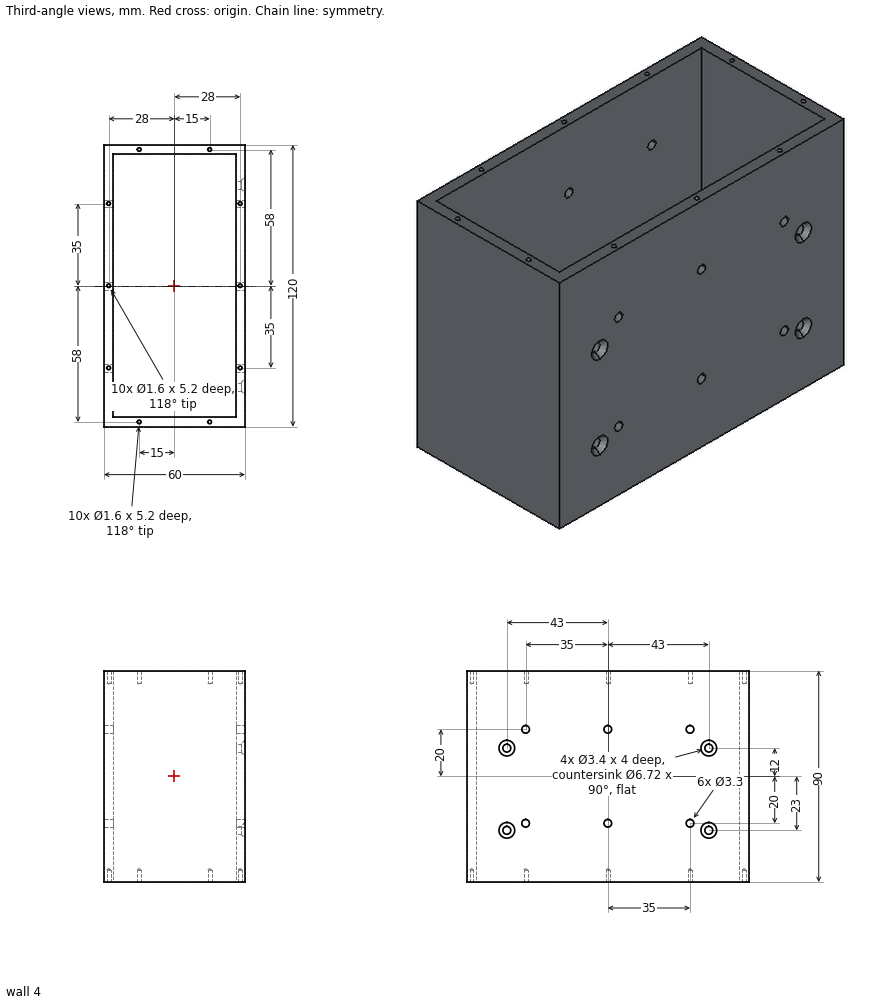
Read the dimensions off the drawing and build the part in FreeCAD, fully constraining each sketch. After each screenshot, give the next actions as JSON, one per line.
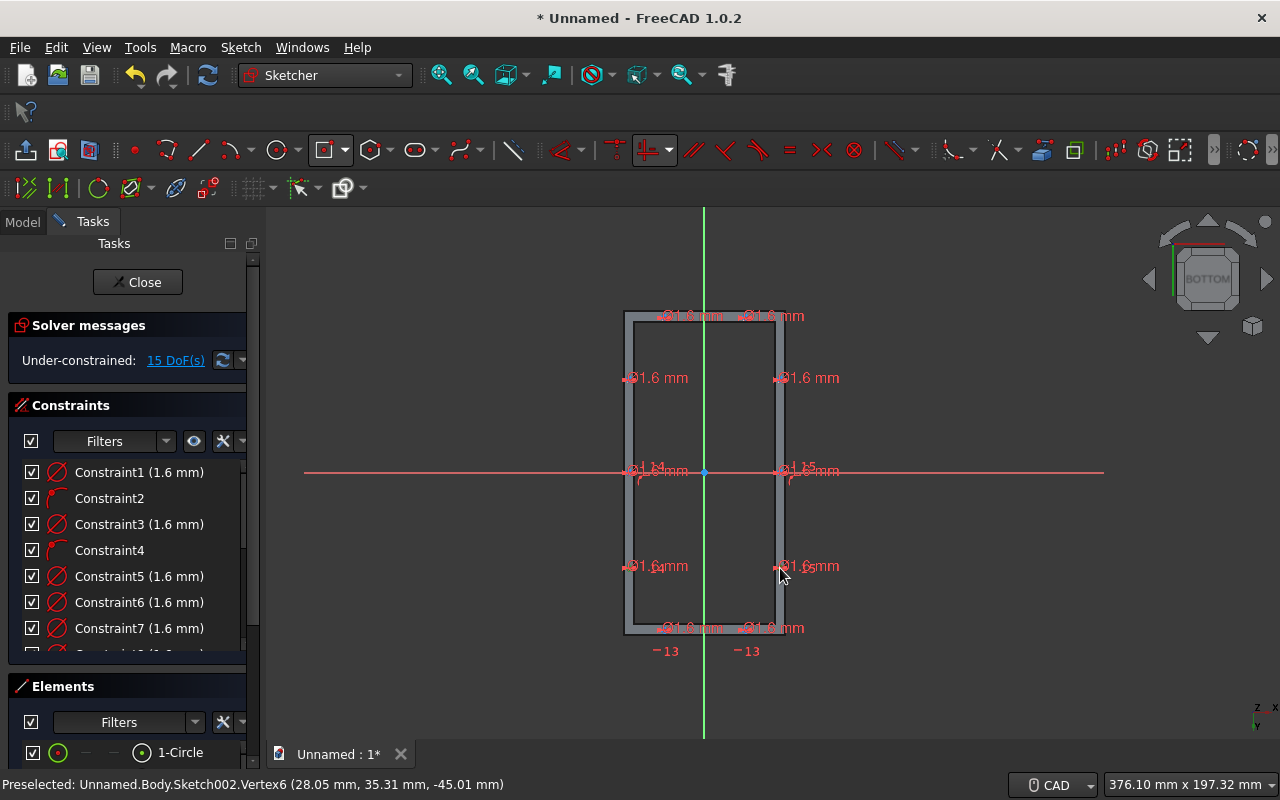
{"action": "left_click", "coordinate": [672, 150]}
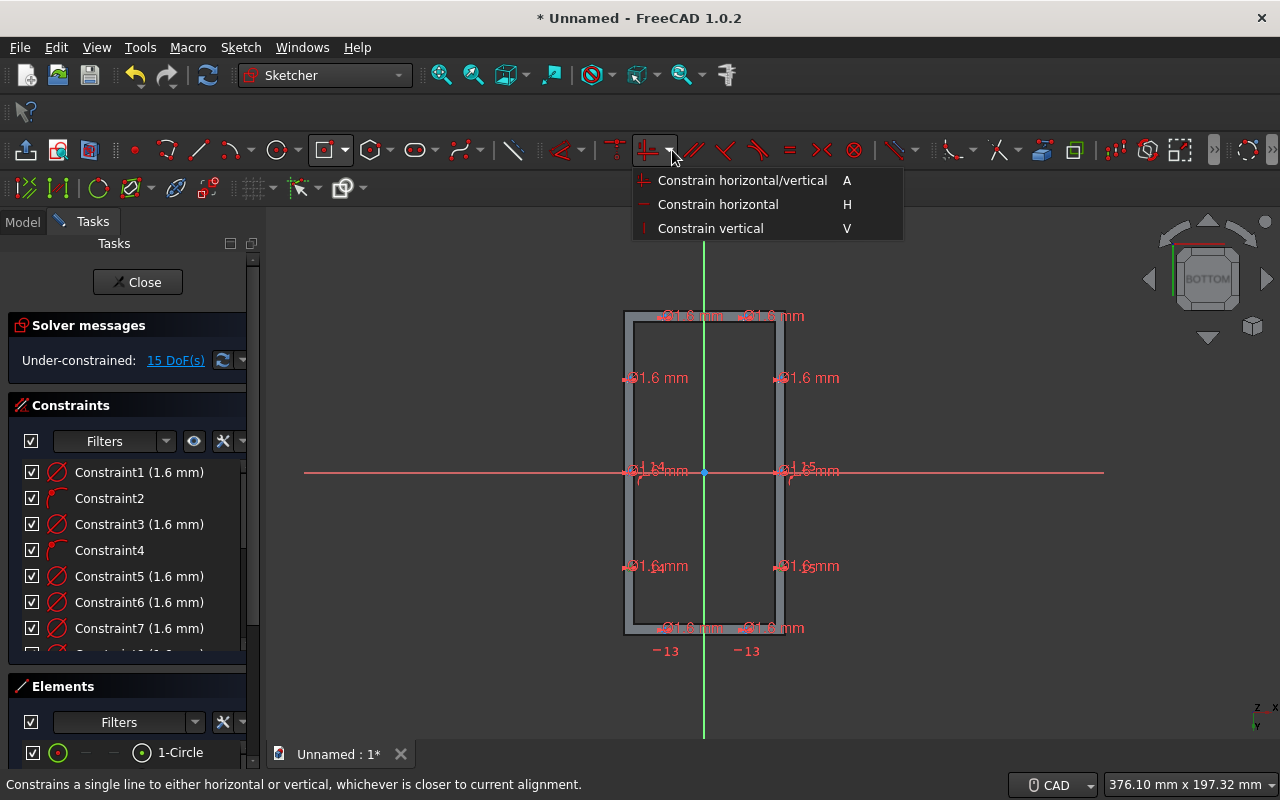
{"action": "left_click", "coordinate": [768, 204]}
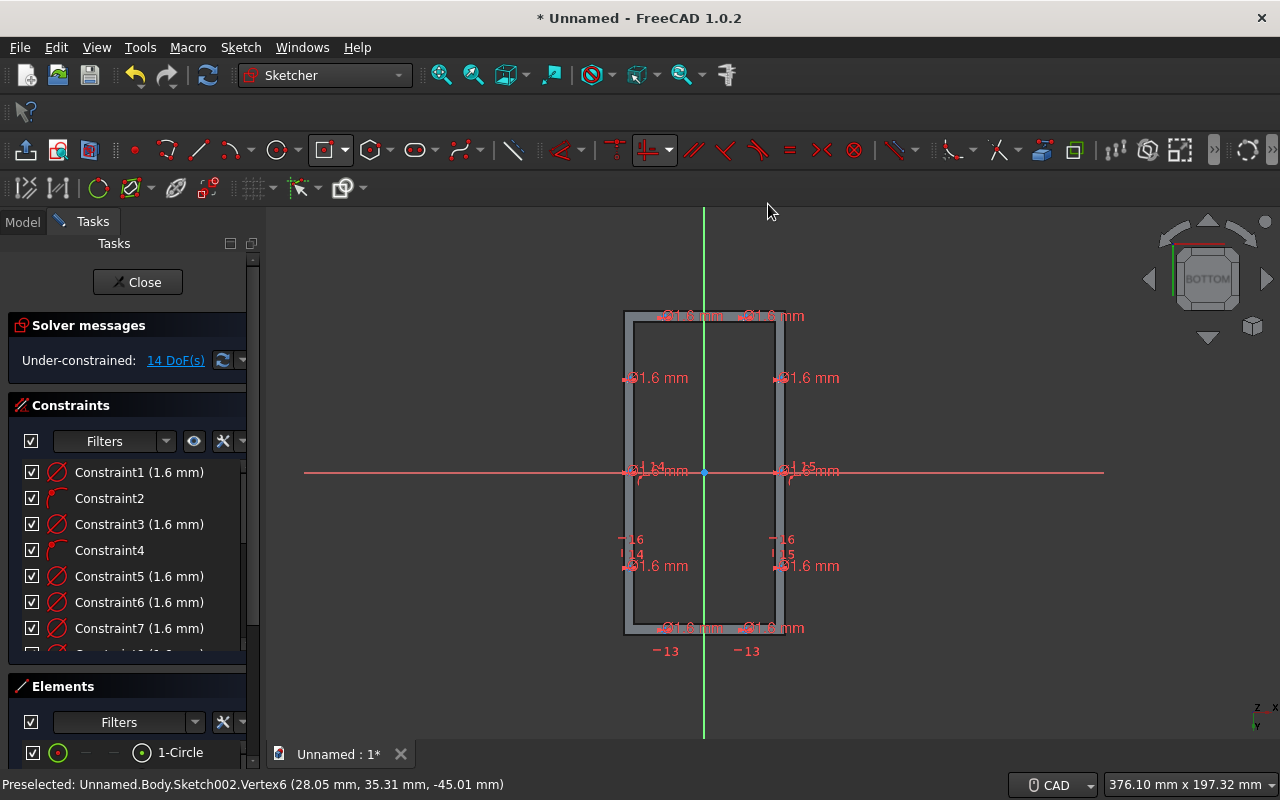
{"action": "left_click", "coordinate": [780, 473]}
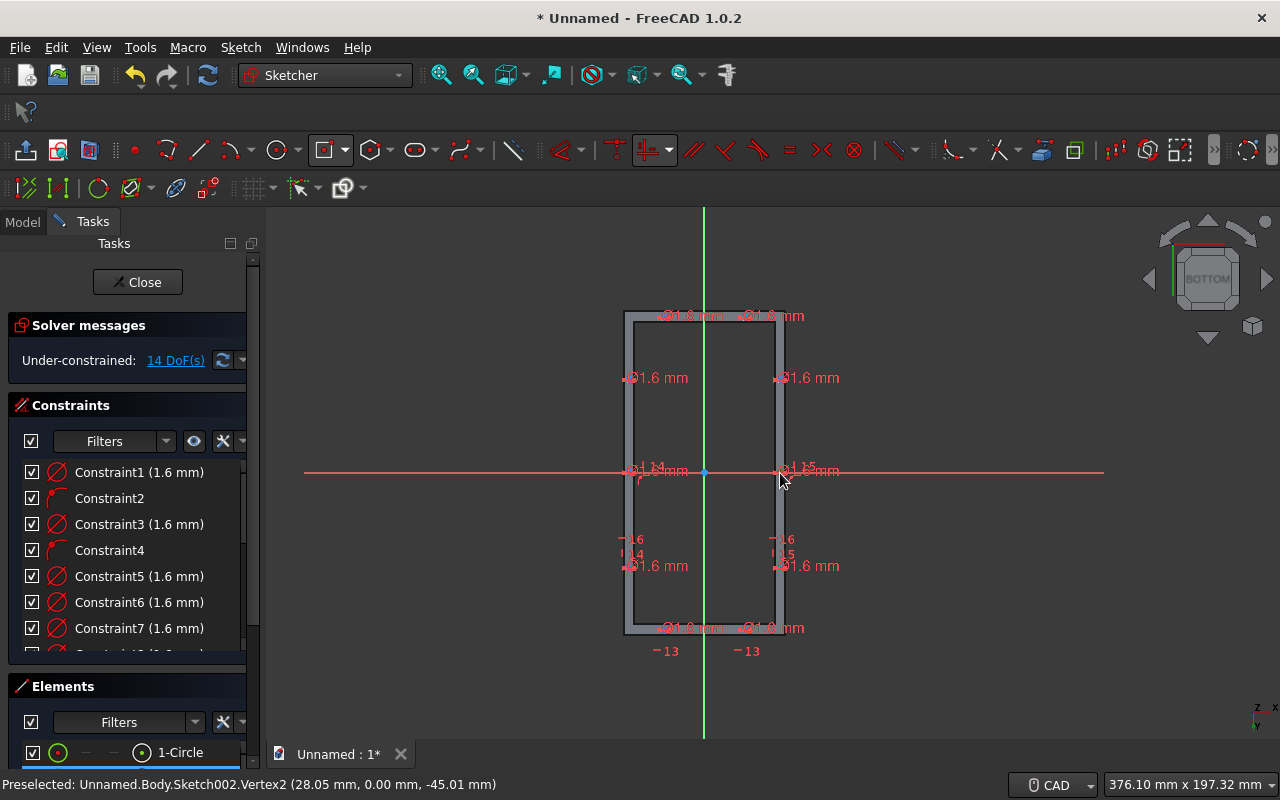
{"action": "left_click", "coordinate": [780, 380]}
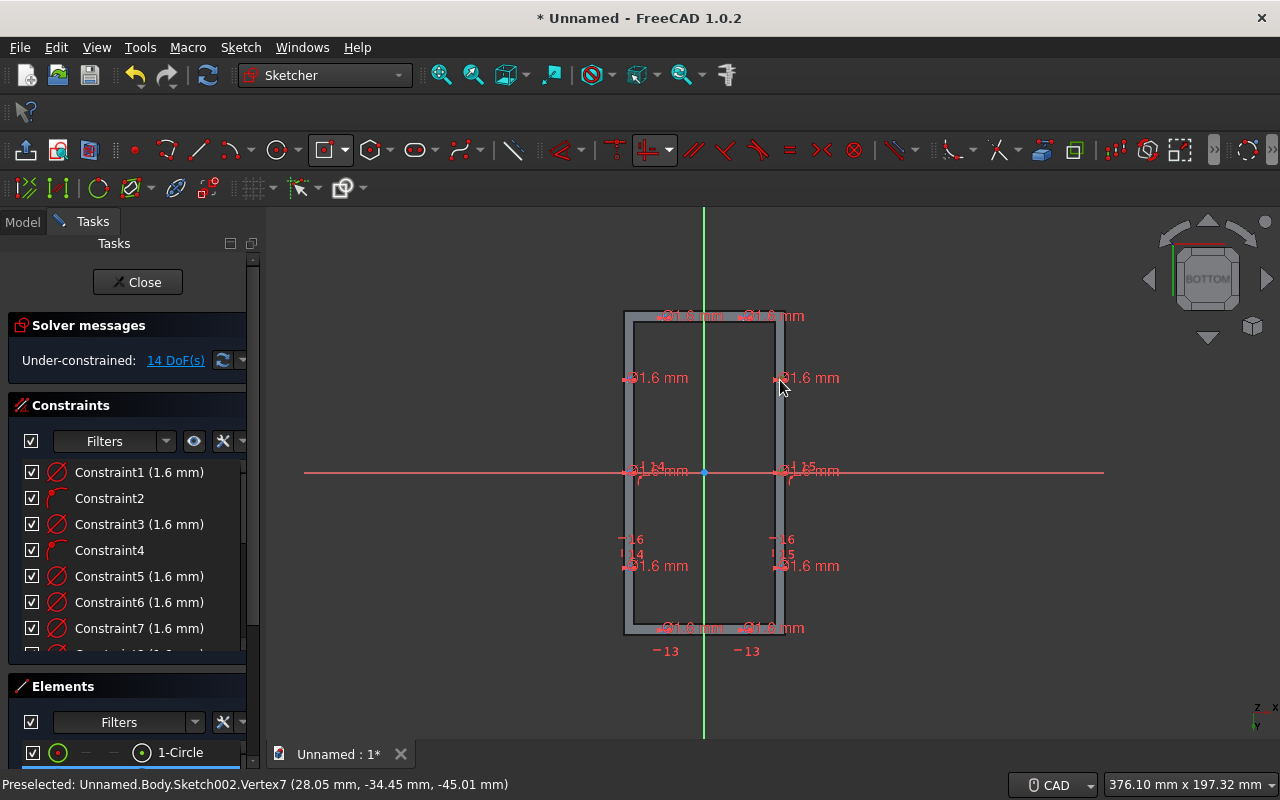
{"action": "left_click", "coordinate": [672, 150]}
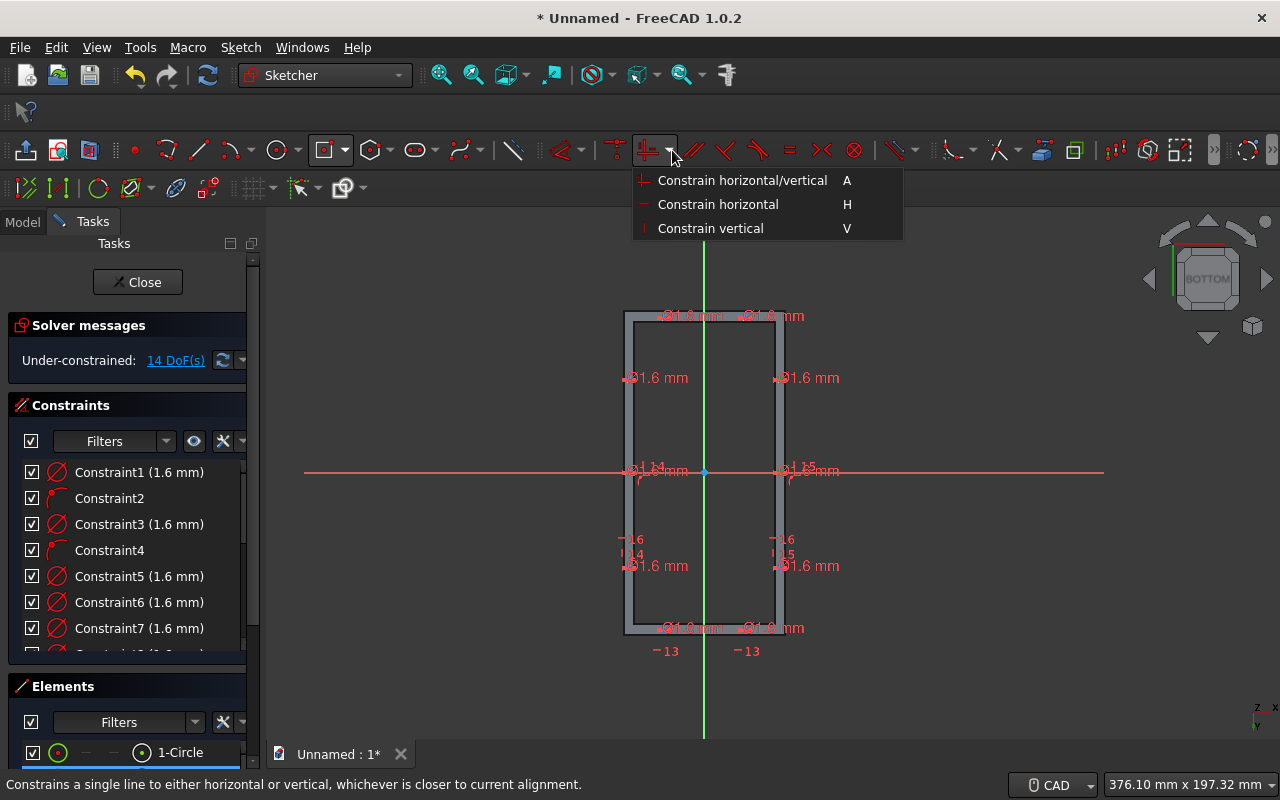
{"action": "left_click", "coordinate": [768, 228]}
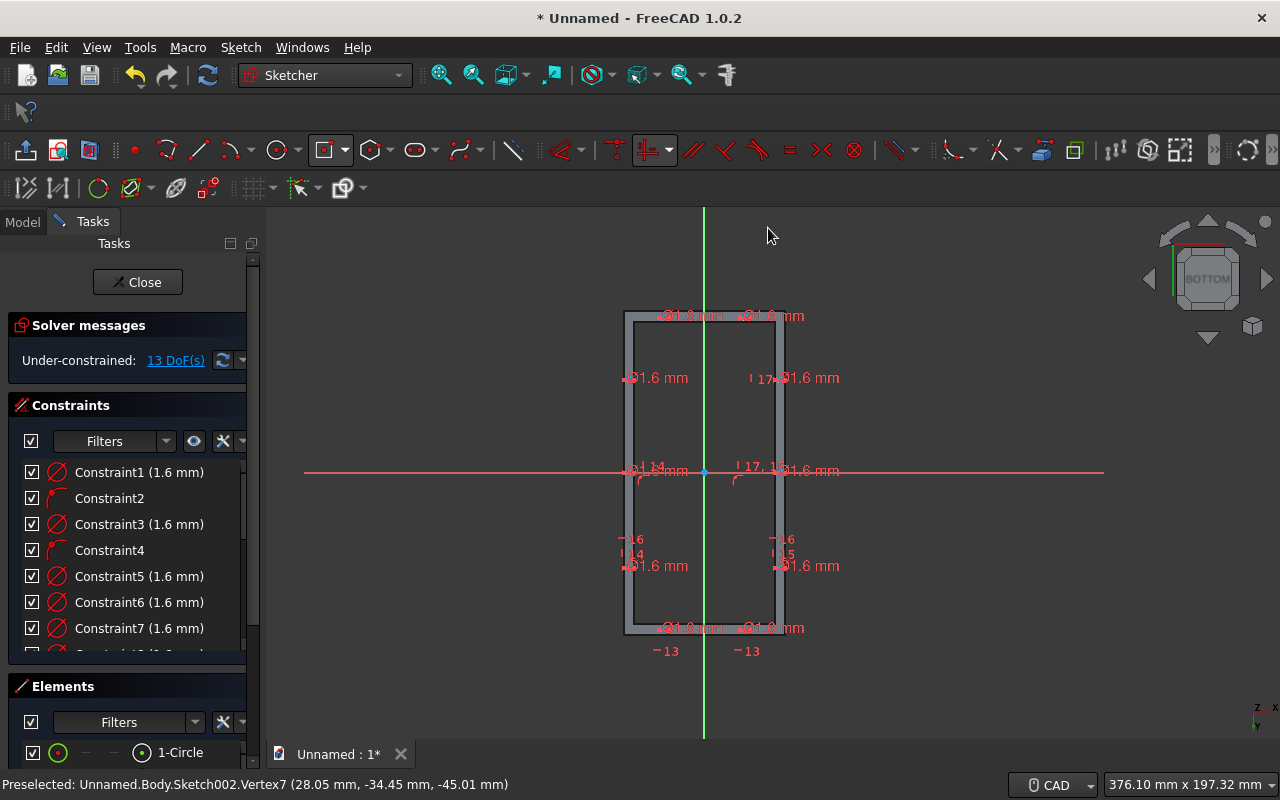
{"action": "left_click", "coordinate": [629, 473]}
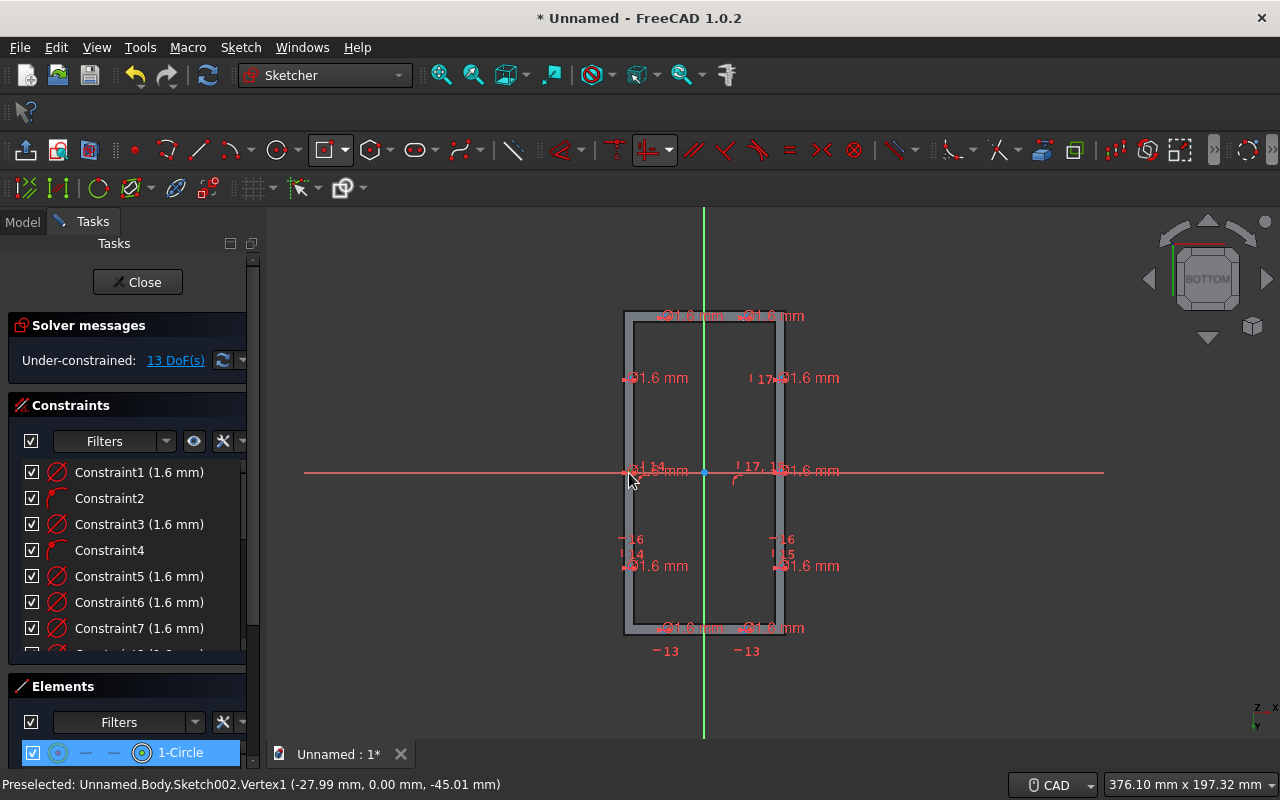
{"action": "left_click", "coordinate": [629, 380]}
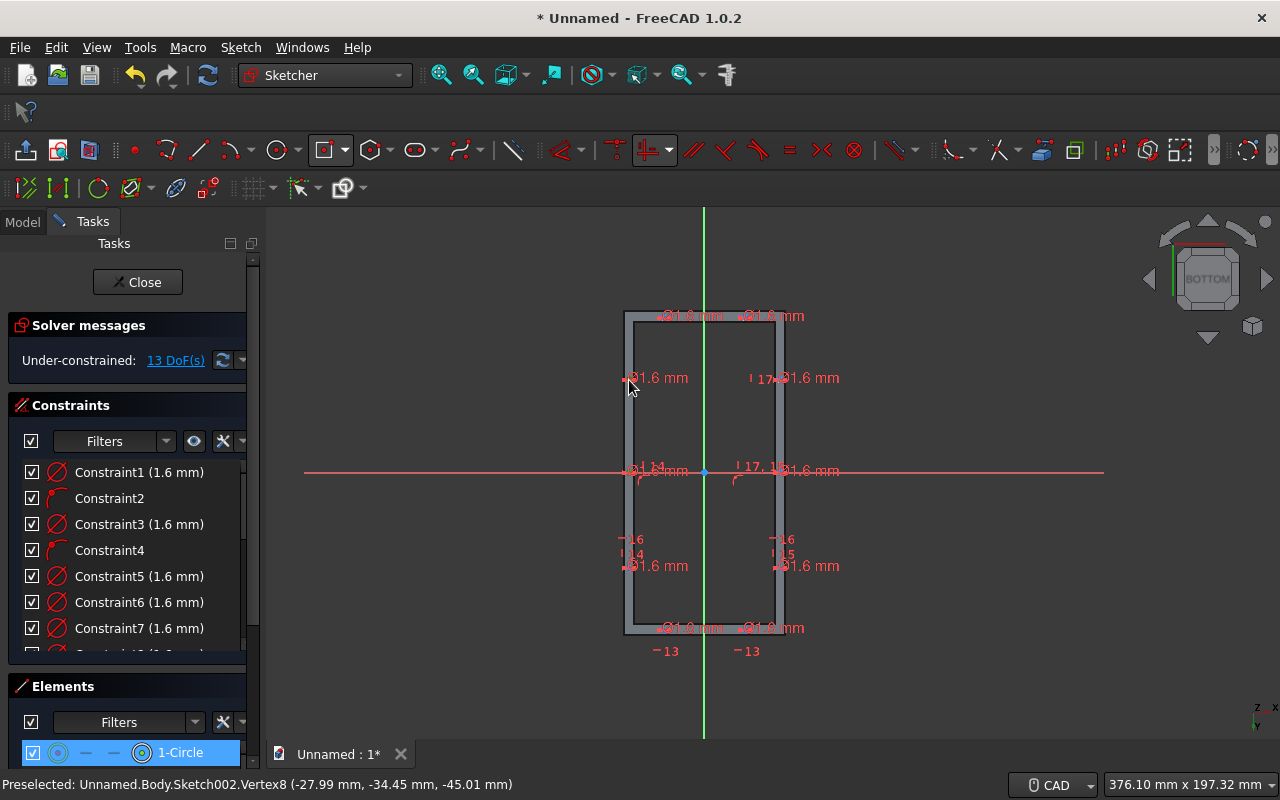
{"action": "left_click", "coordinate": [672, 150]}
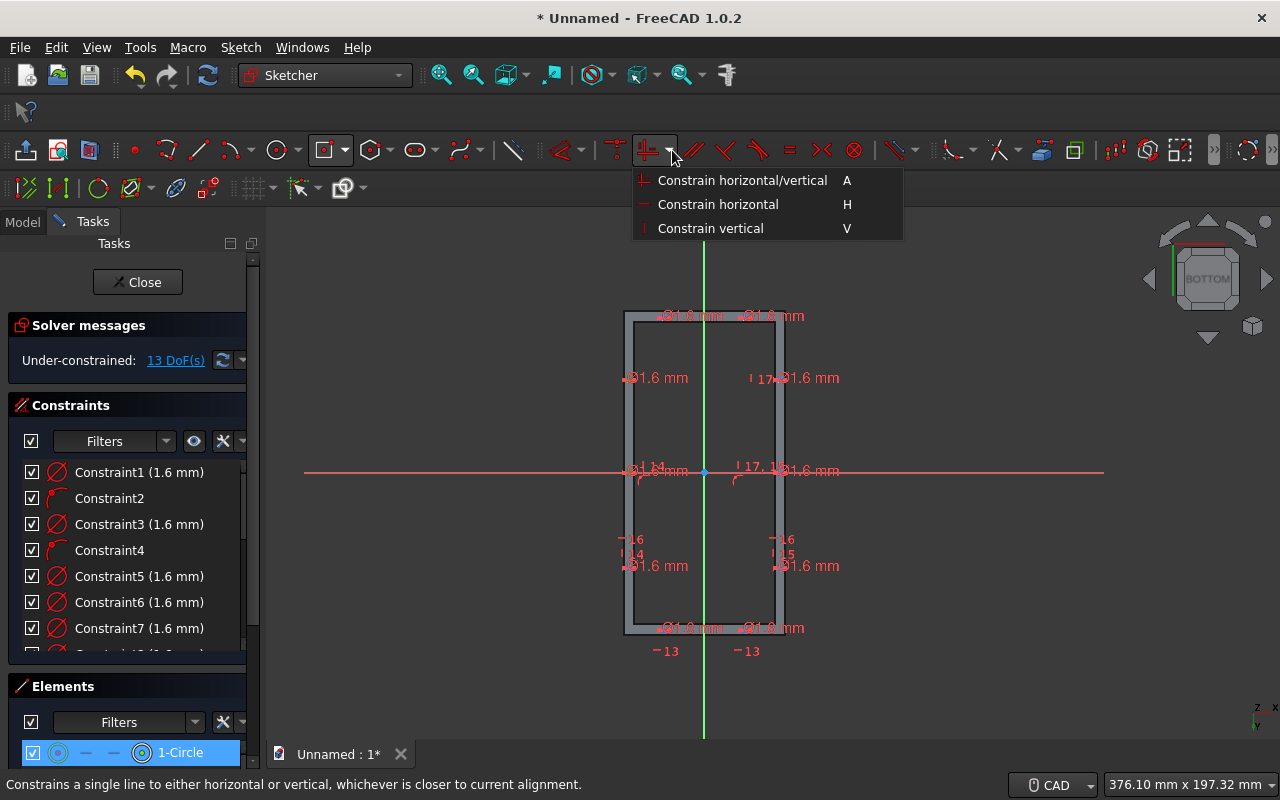
{"action": "left_click", "coordinate": [768, 228]}